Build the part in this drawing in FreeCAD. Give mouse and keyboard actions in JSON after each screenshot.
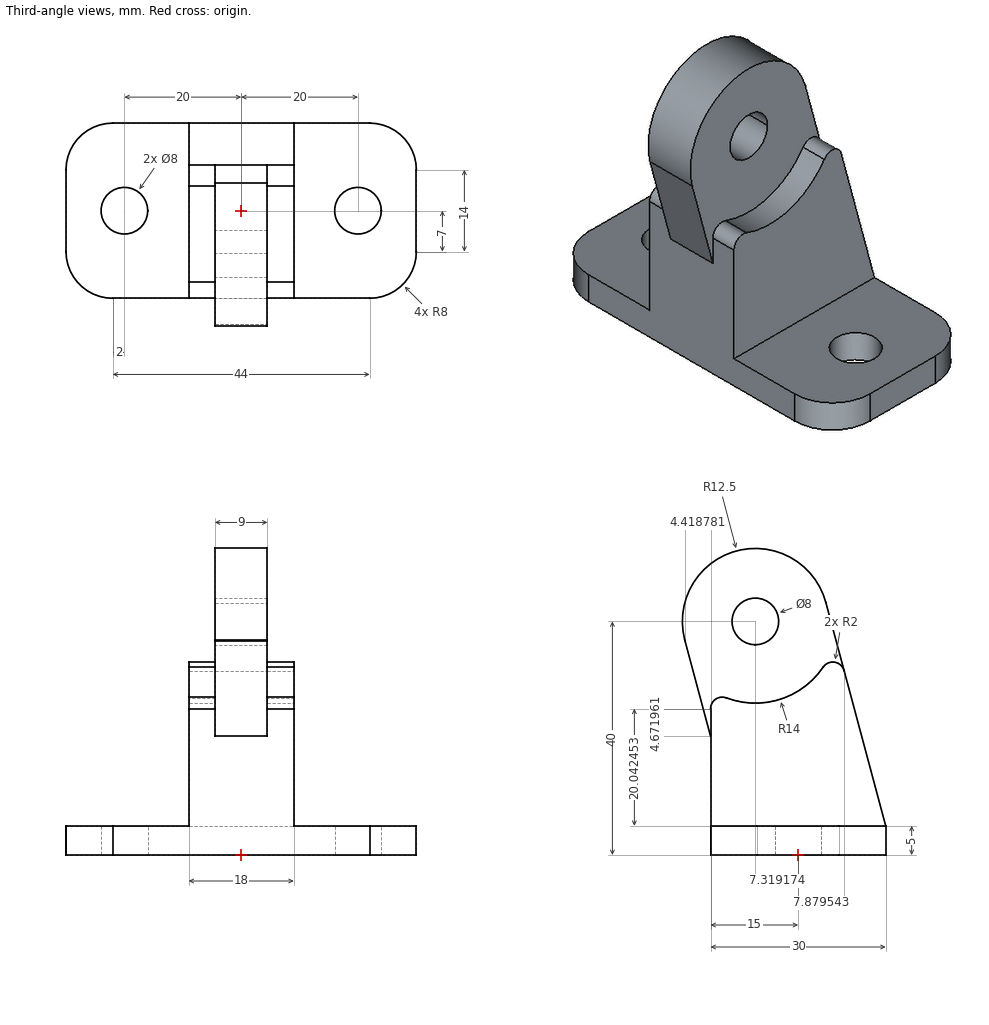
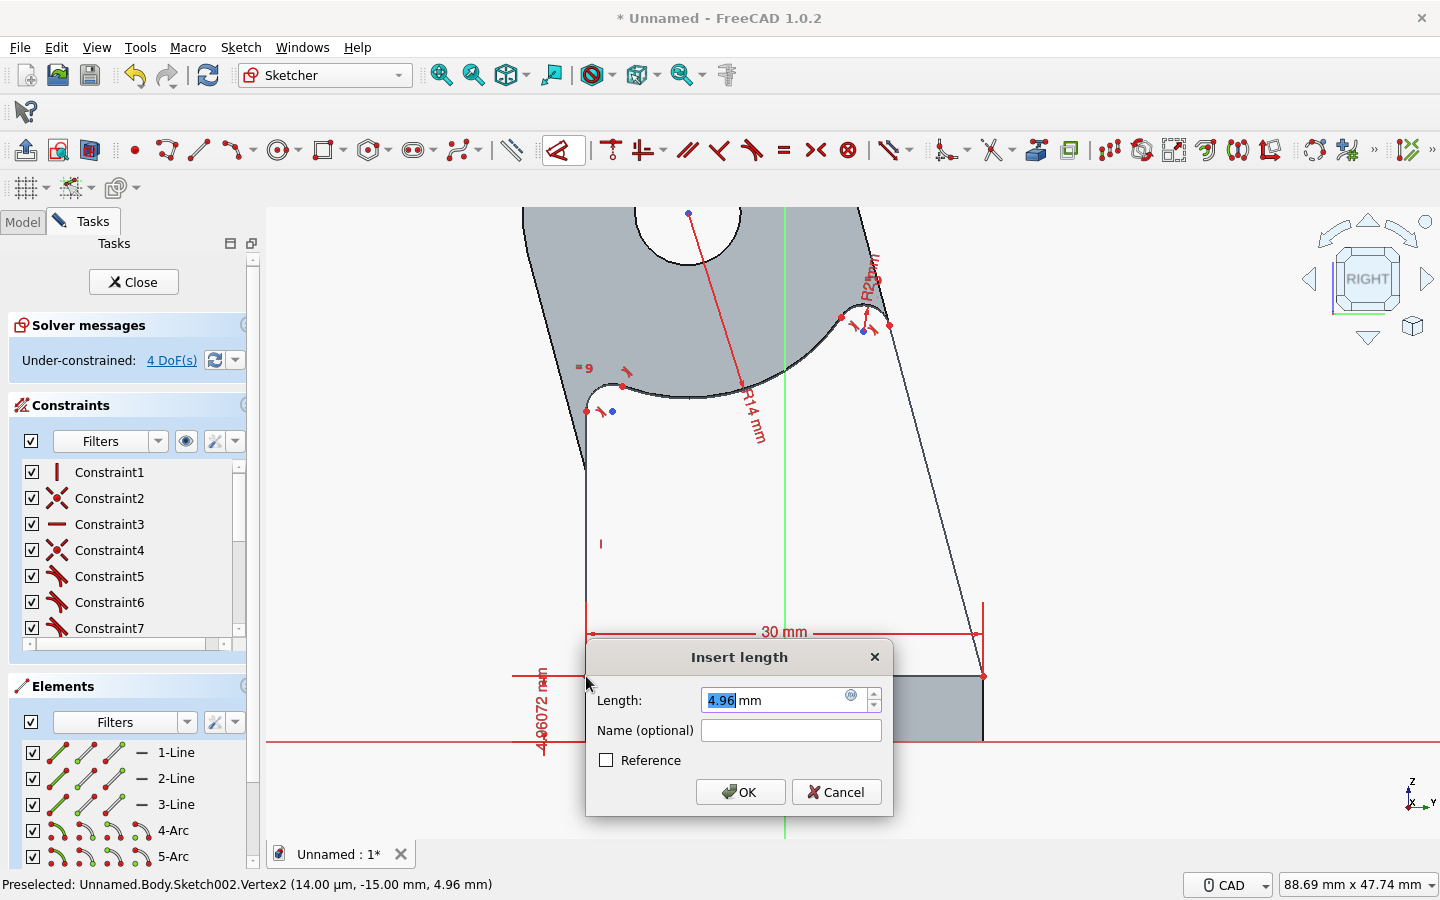
{"action": "type", "text": "5"}
{"action": "key", "text": "Return"}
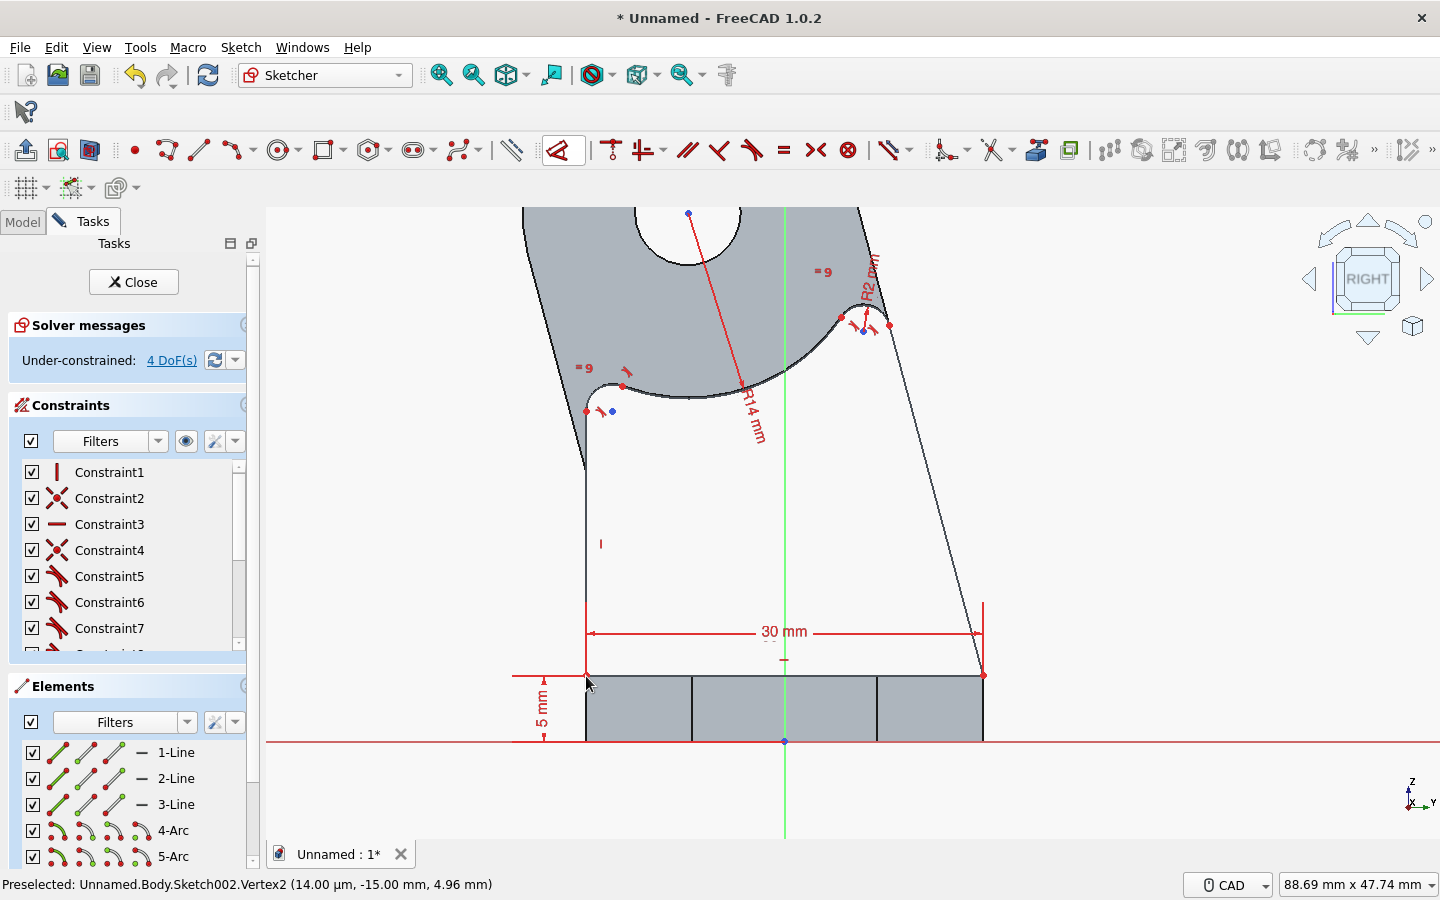
{"action": "left_click", "coordinate": [586, 411]}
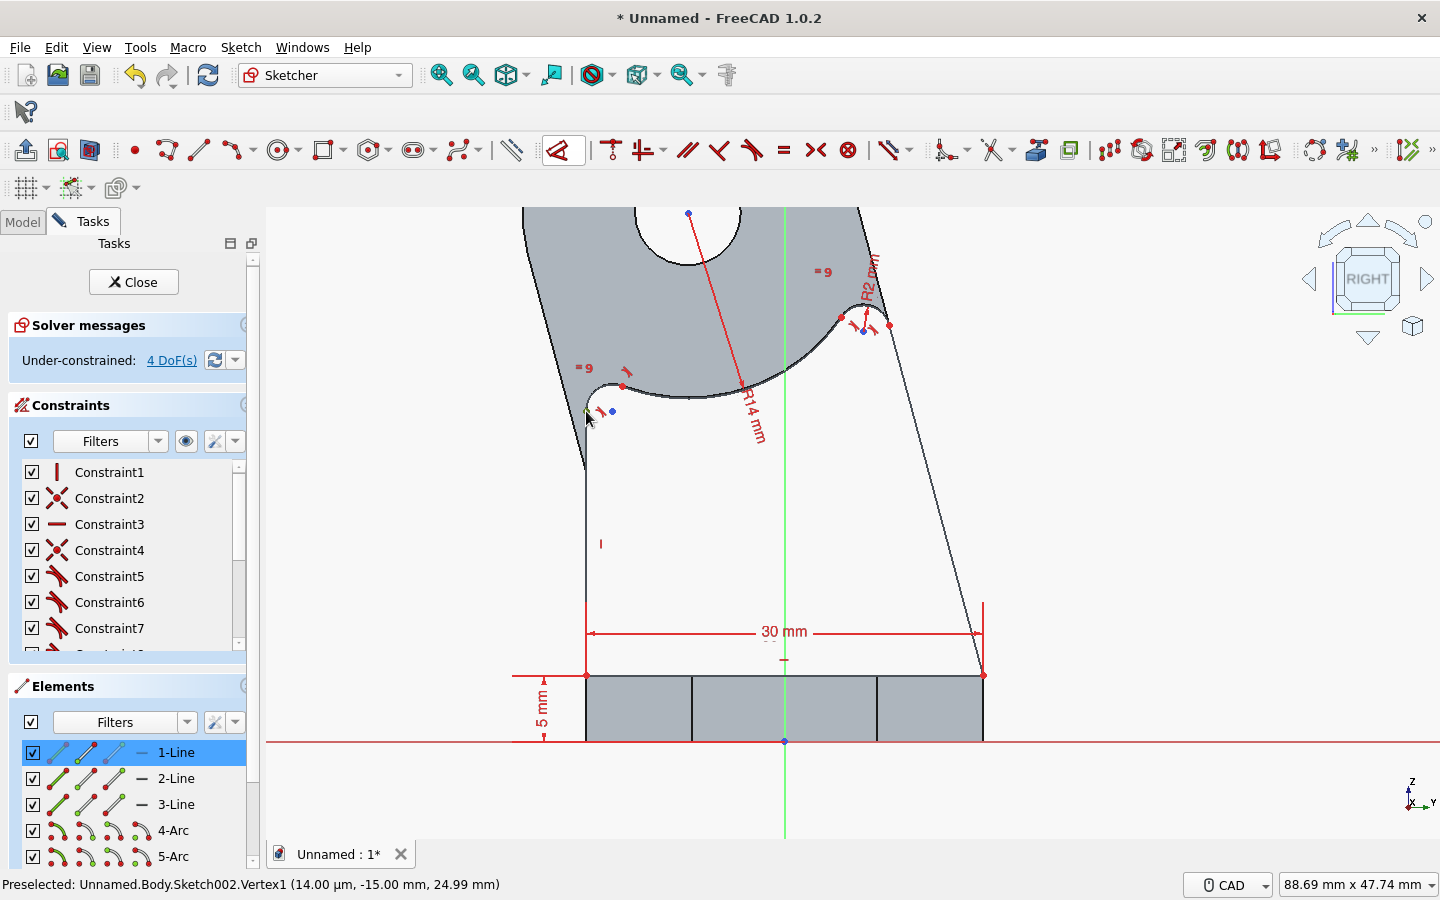
{"action": "key", "text": "l"}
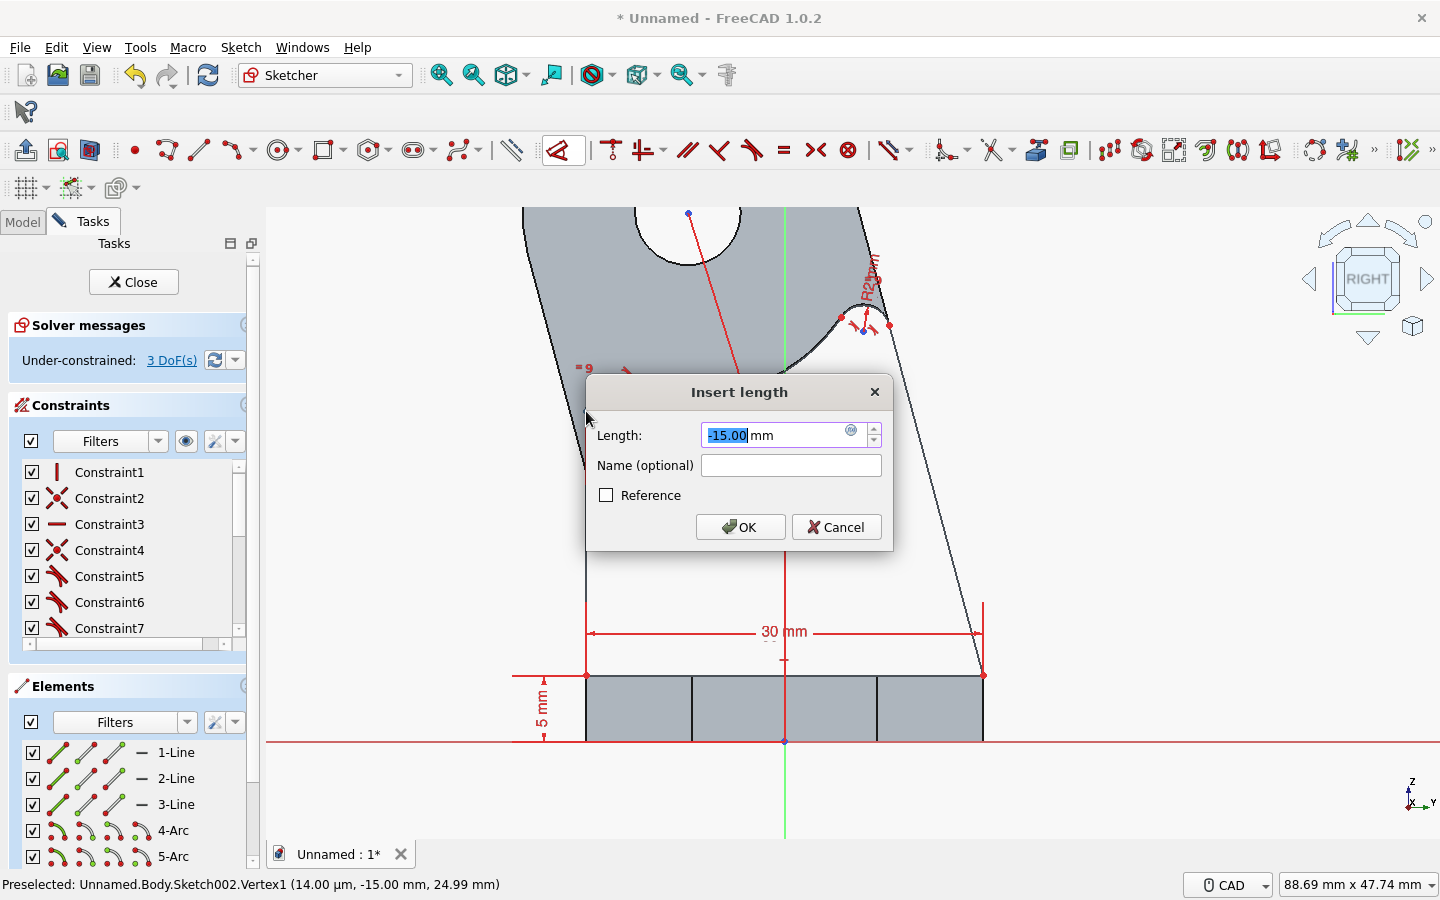
{"action": "type", "text": "-15"}
{"action": "key", "text": "Return"}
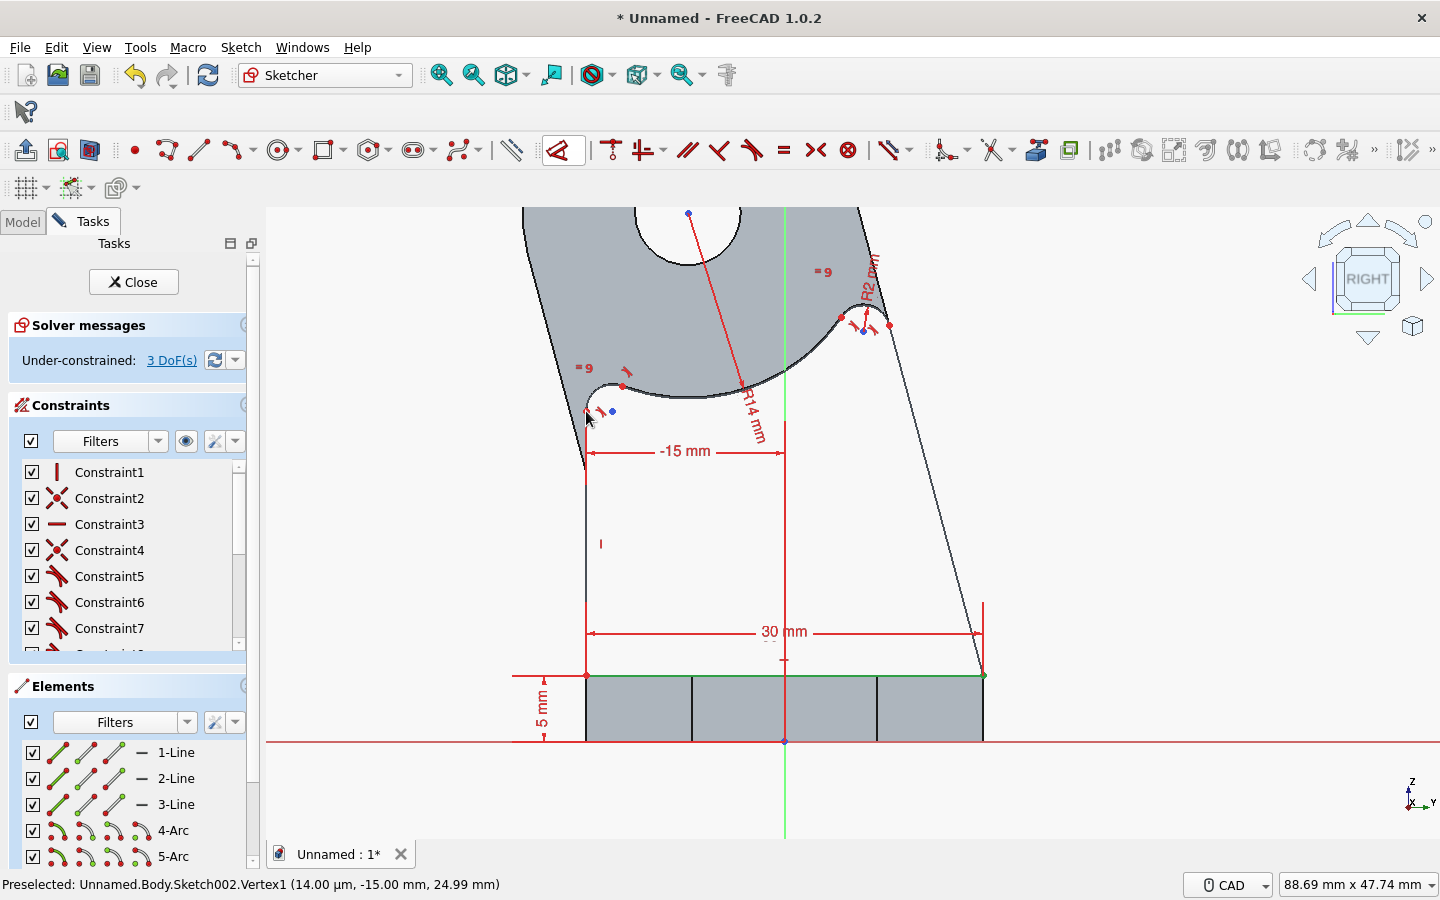
{"action": "scroll", "coordinate": [783, 728], "scroll_direction": "down", "scroll_amount": 1}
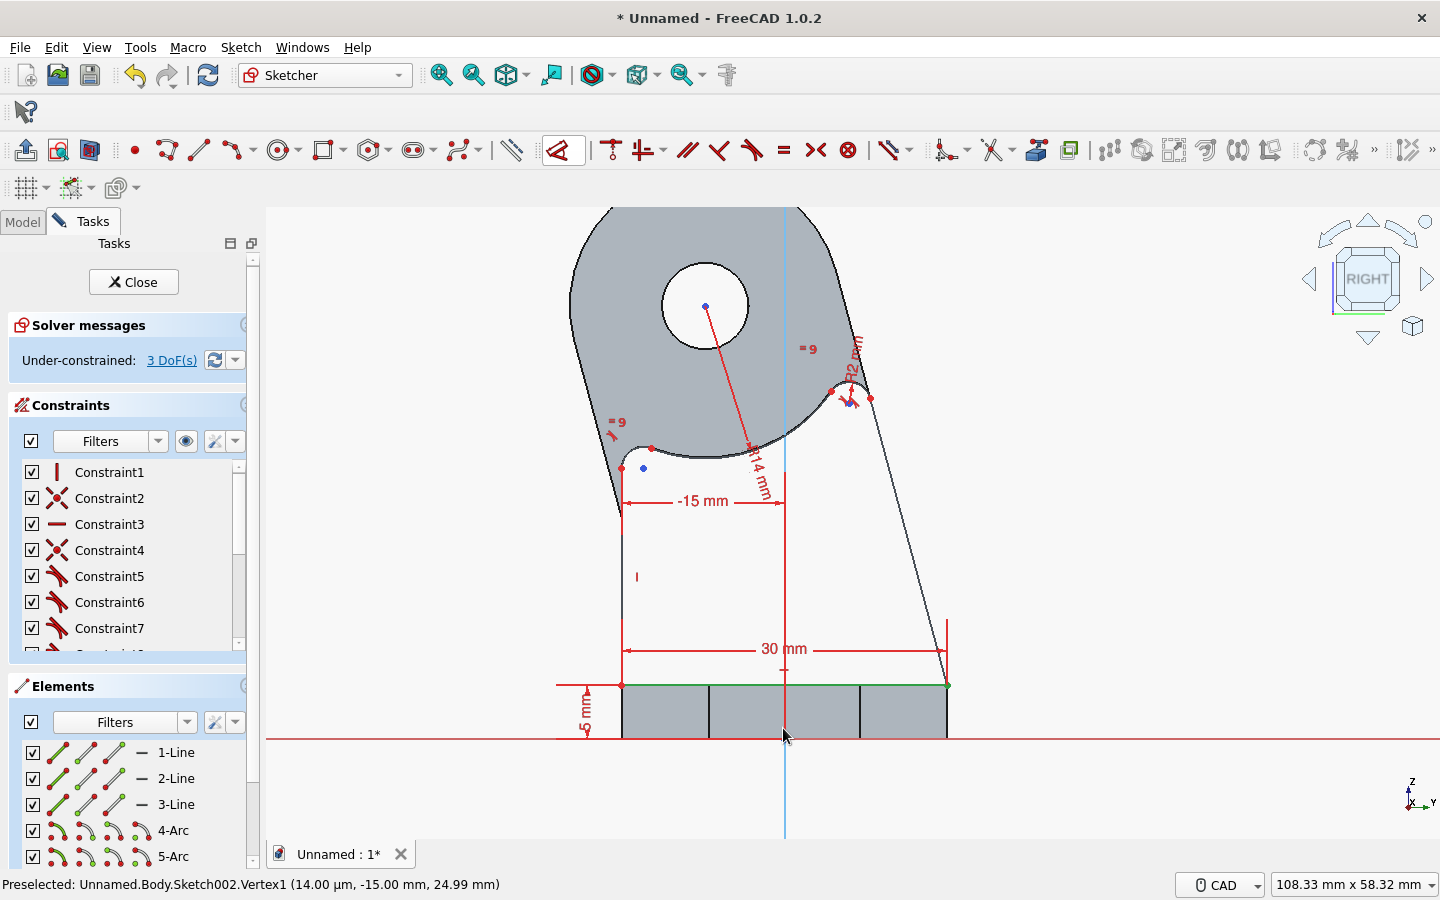
{"action": "left_click", "coordinate": [706, 307]}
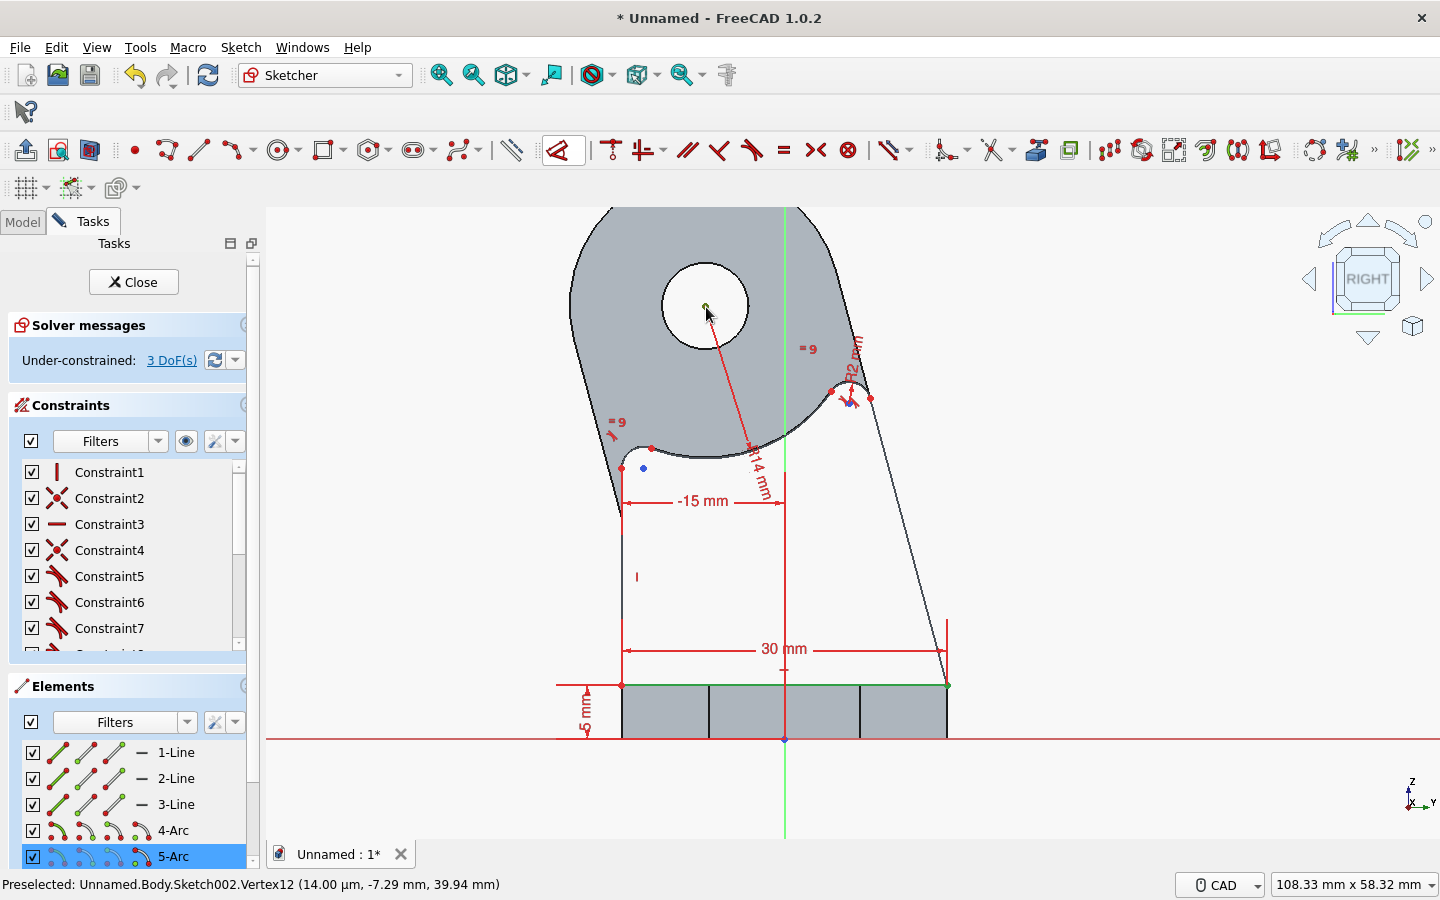
{"action": "key", "text": "i"}